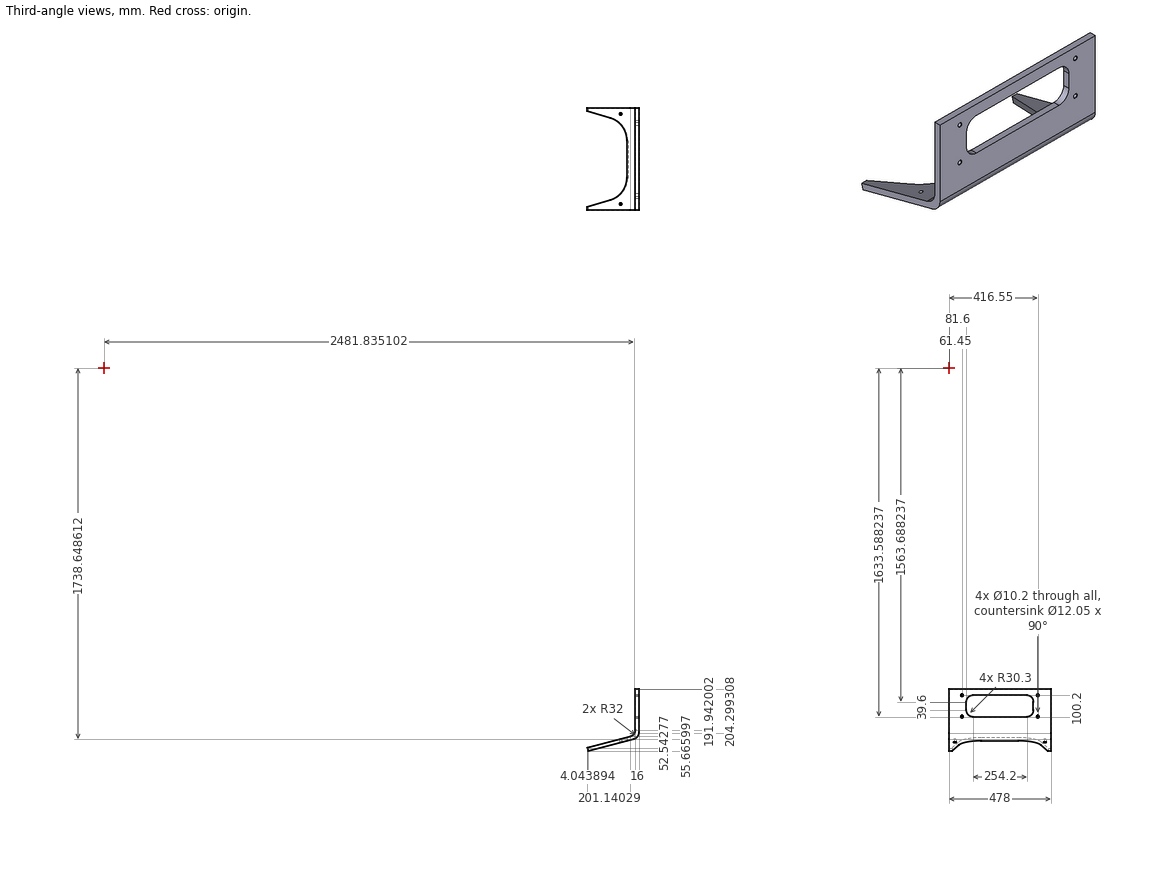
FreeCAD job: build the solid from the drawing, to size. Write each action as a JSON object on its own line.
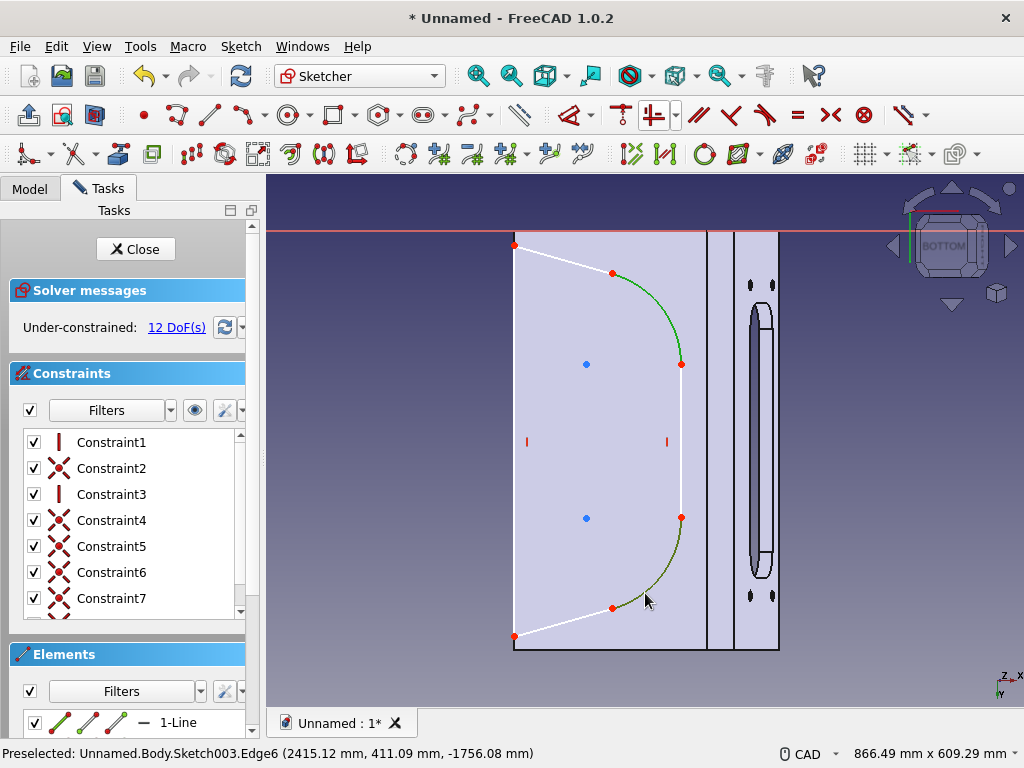
{"action": "left_click", "coordinate": [798, 116]}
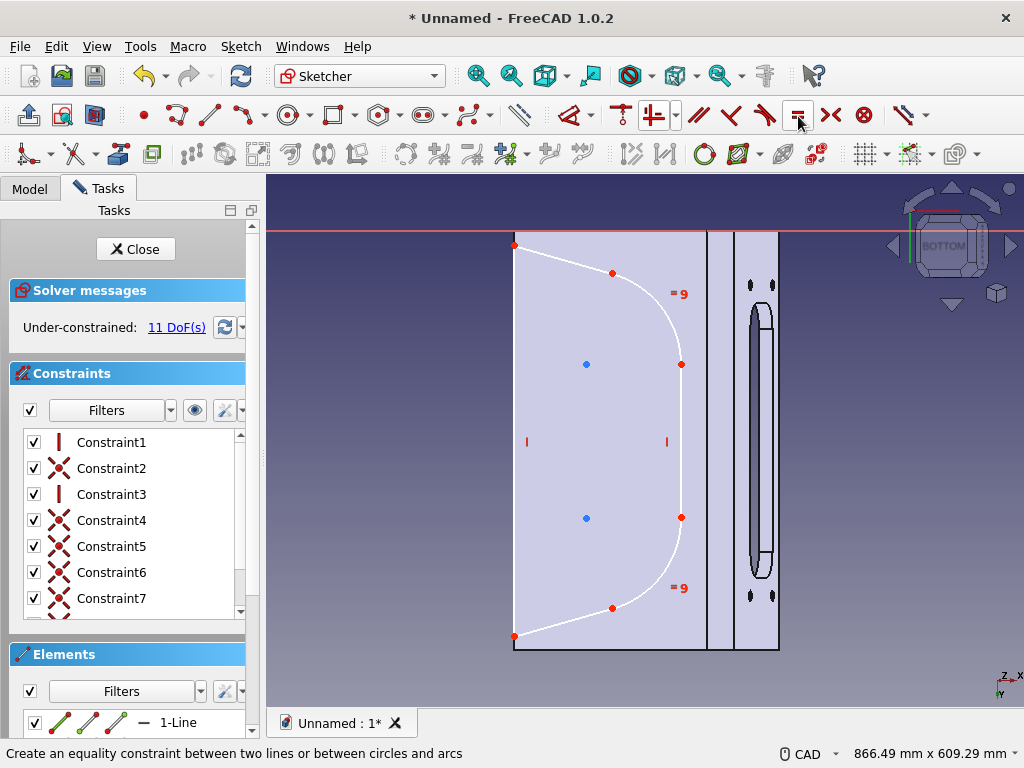
{"action": "left_click", "coordinate": [568, 116]}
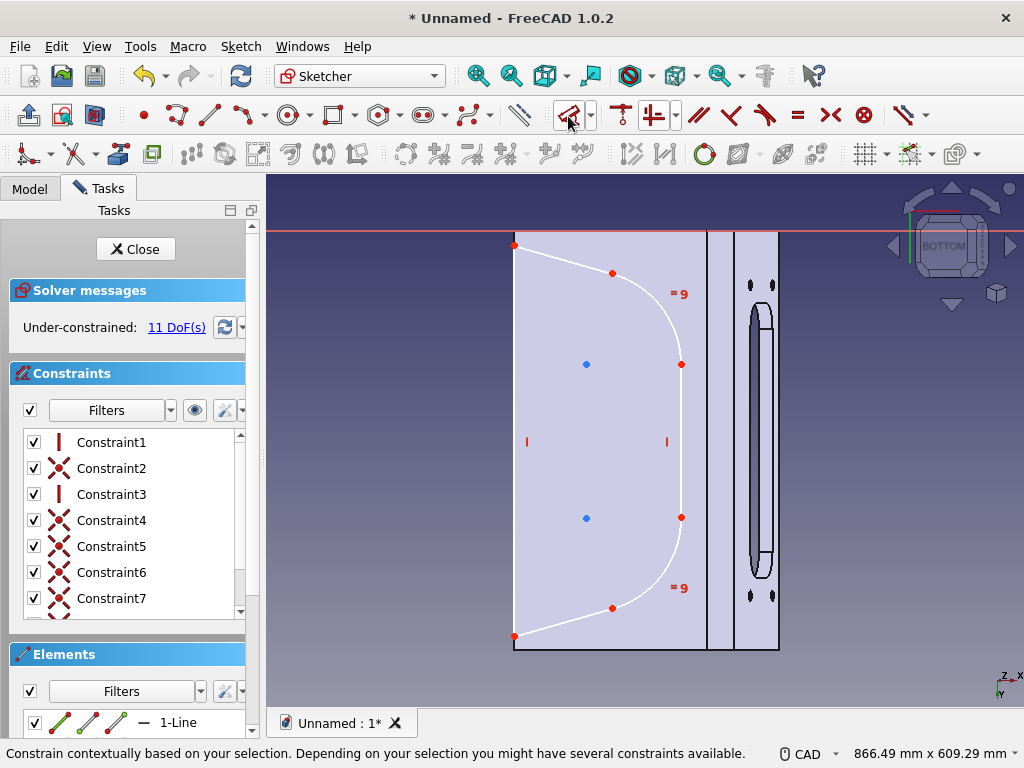
{"action": "left_click", "coordinate": [674, 329]}
{"action": "left_click", "coordinate": [704, 317]}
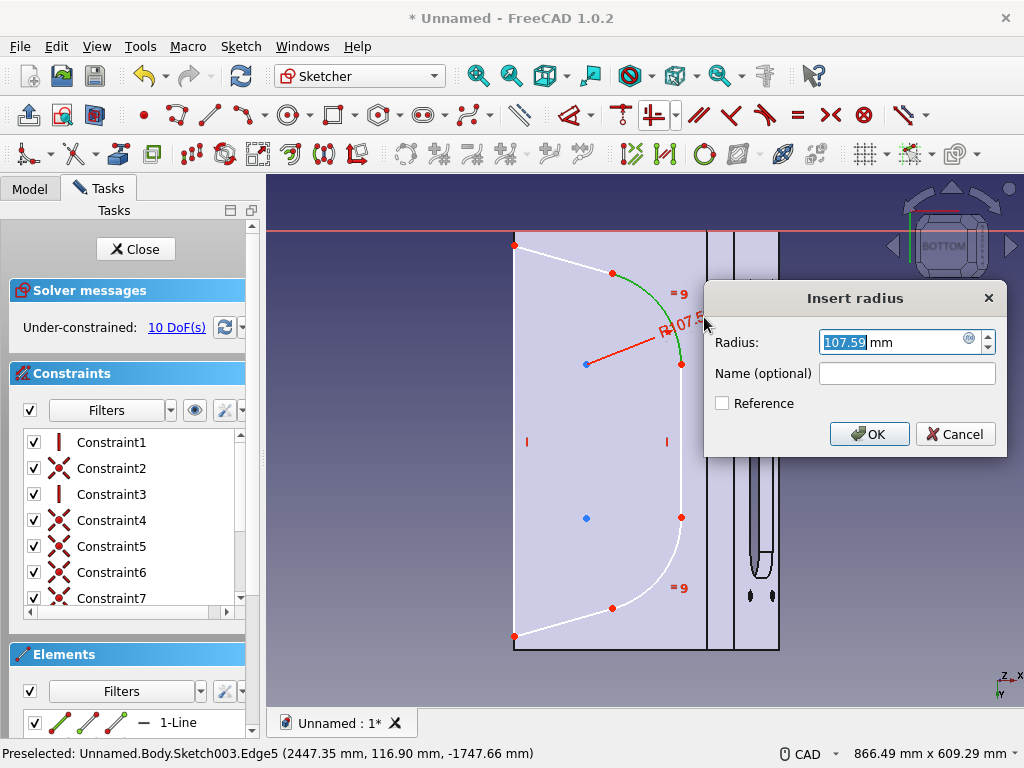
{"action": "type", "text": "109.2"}
{"action": "key", "text": "Return"}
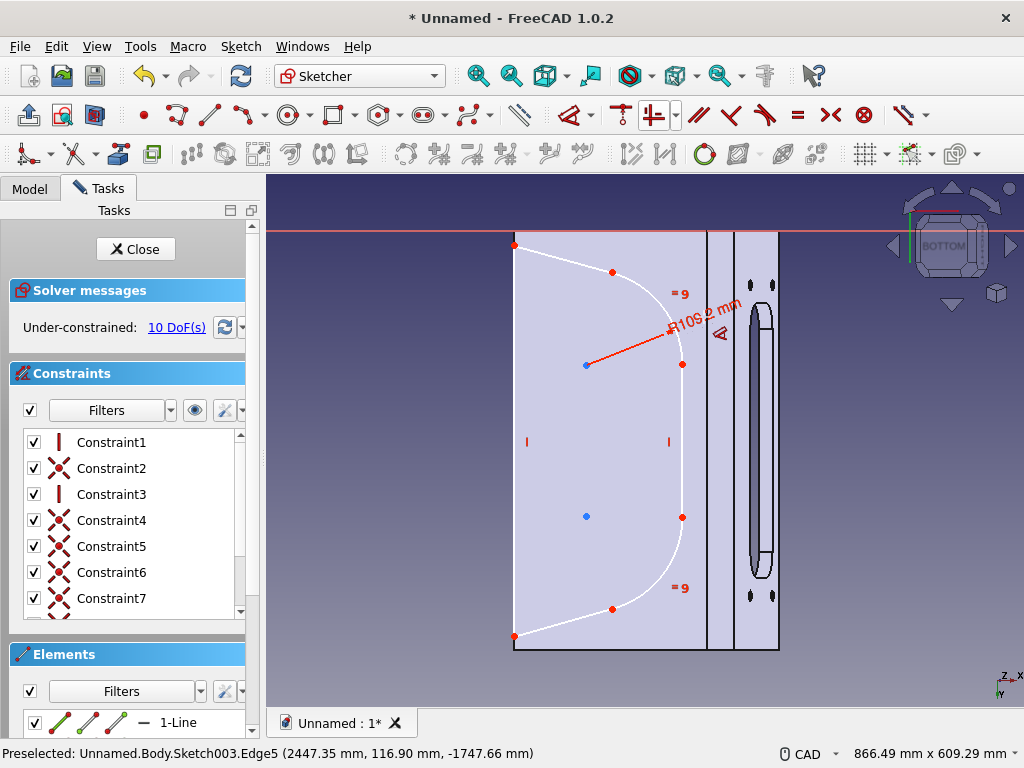
{"action": "left_click", "coordinate": [514, 363]}
{"action": "left_click", "coordinate": [480, 442]}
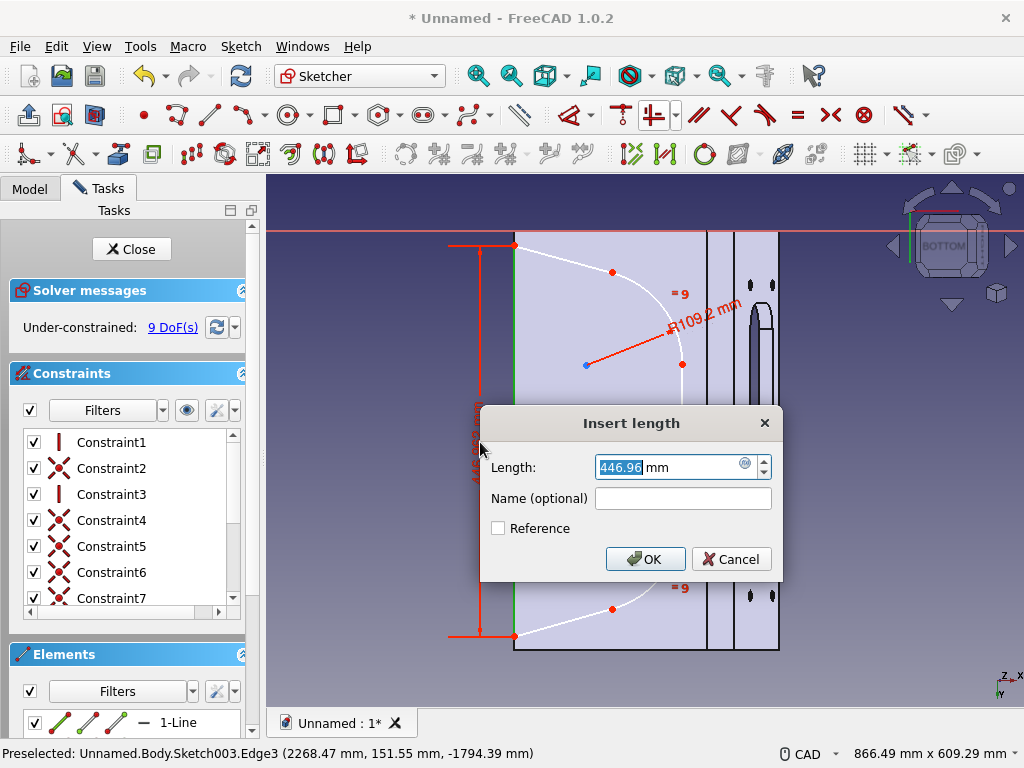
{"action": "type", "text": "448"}
{"action": "key", "text": "Return"}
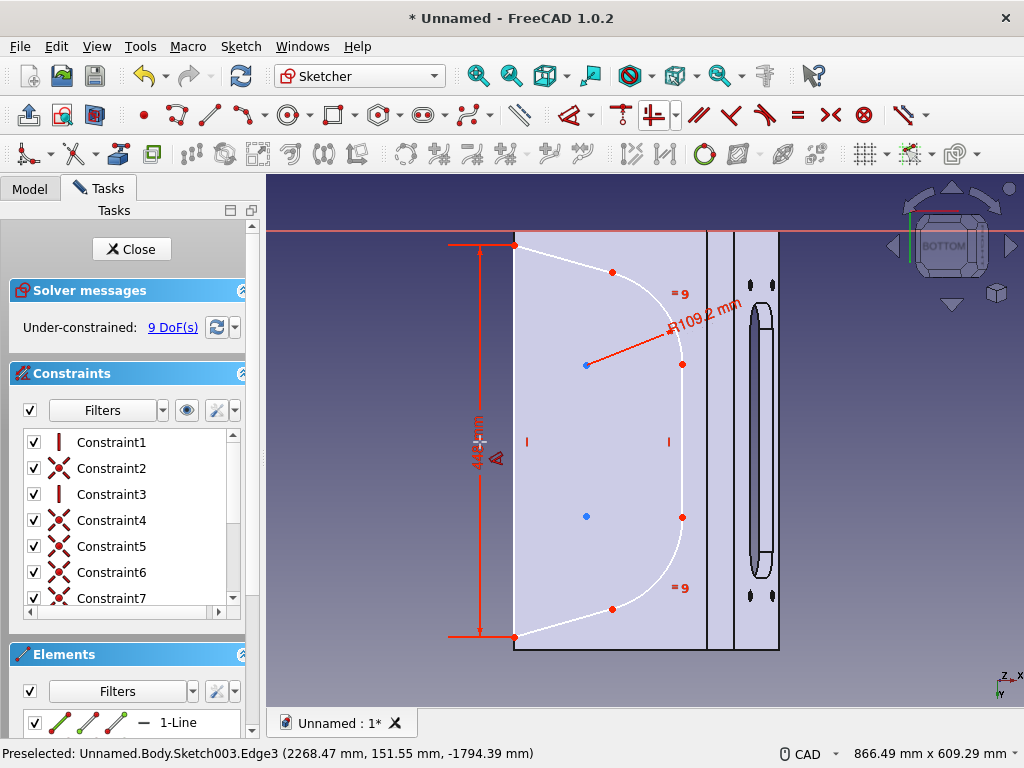
{"action": "scroll", "coordinate": [514, 245], "scroll_direction": "up", "scroll_amount": 6}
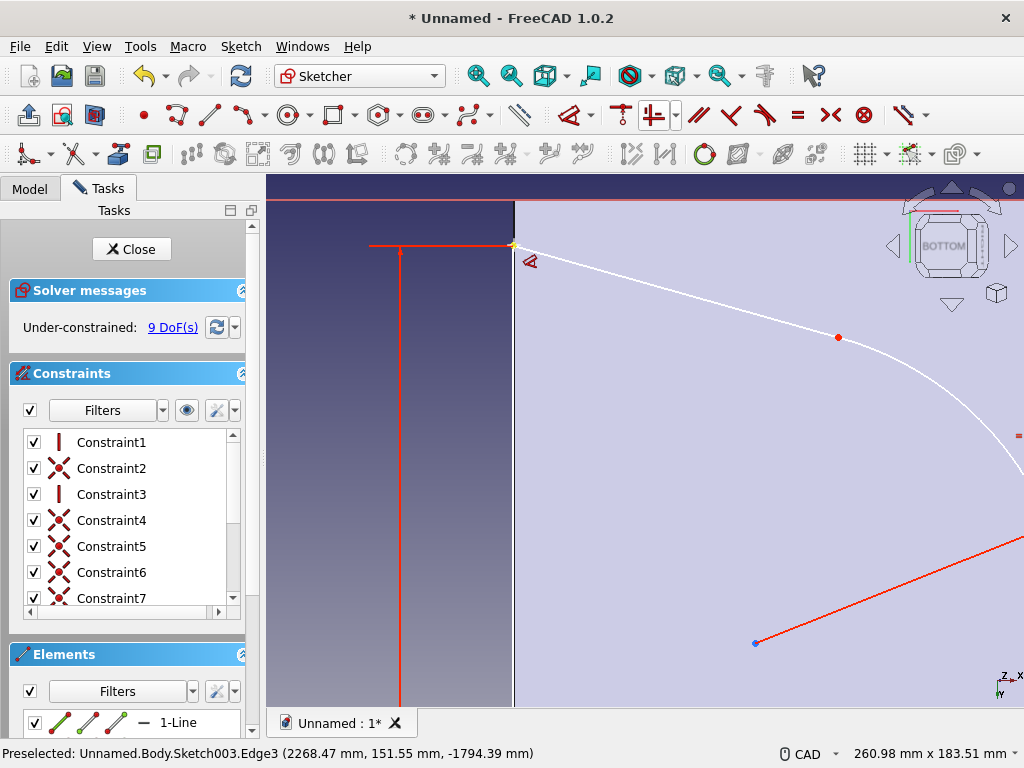
{"action": "left_click", "coordinate": [513, 246]}
{"action": "left_click", "coordinate": [547, 224]}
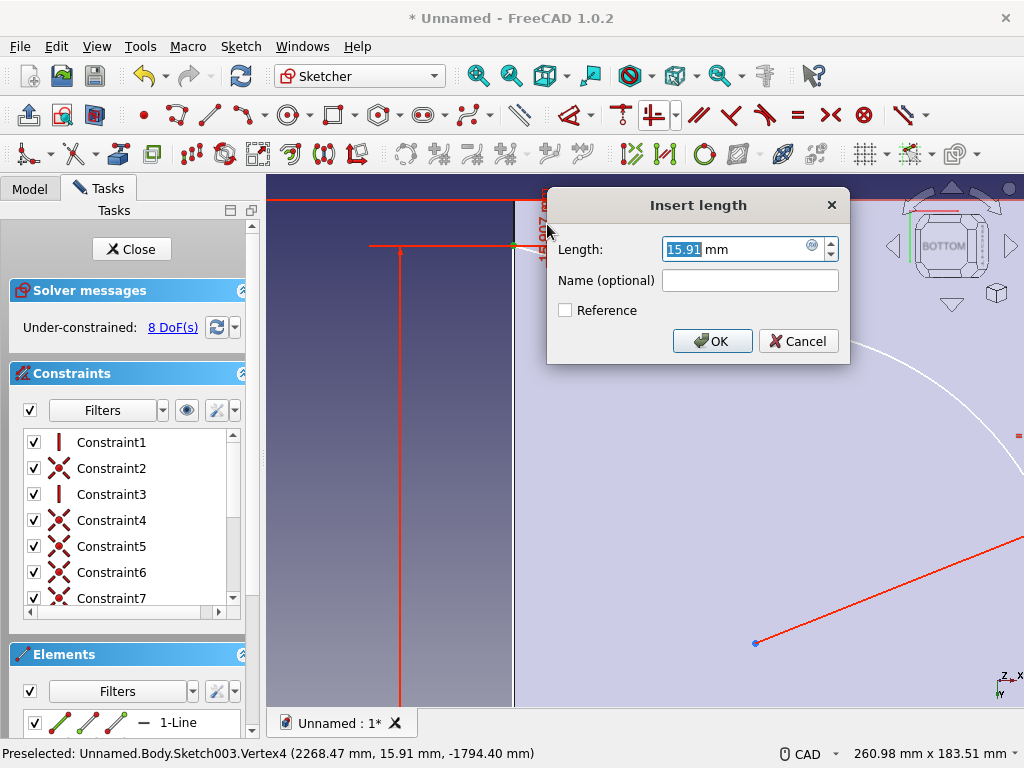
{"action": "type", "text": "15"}
{"action": "key", "text": "Return"}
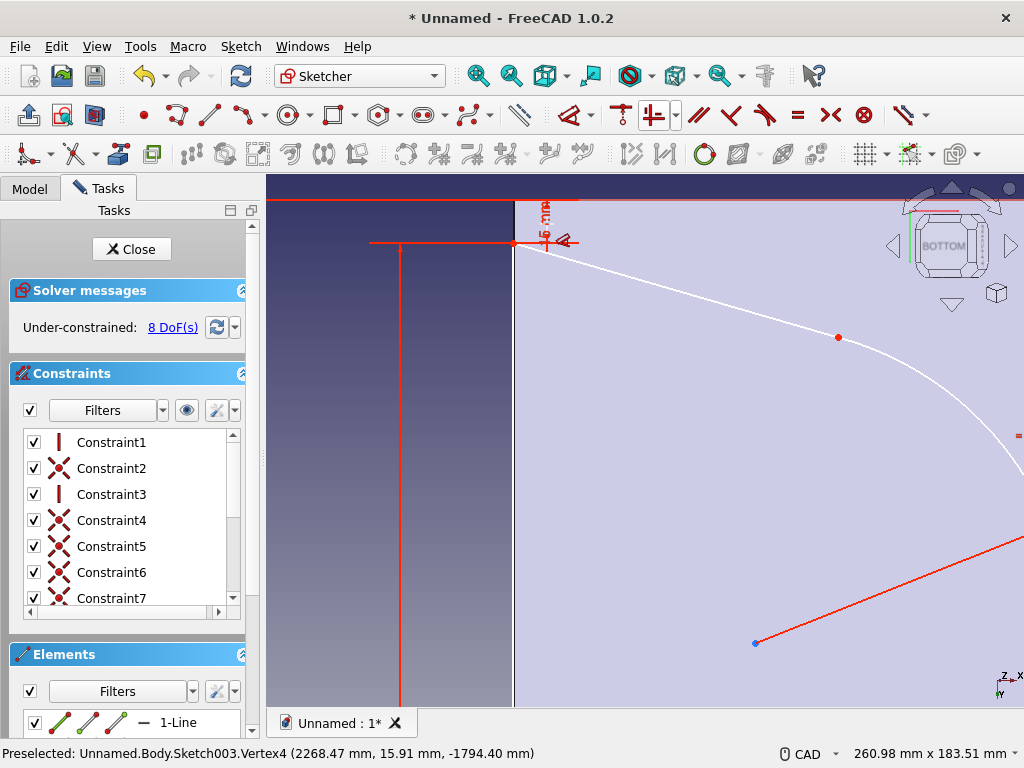
{"action": "scroll", "coordinate": [506, 292], "scroll_direction": "down", "scroll_amount": 7}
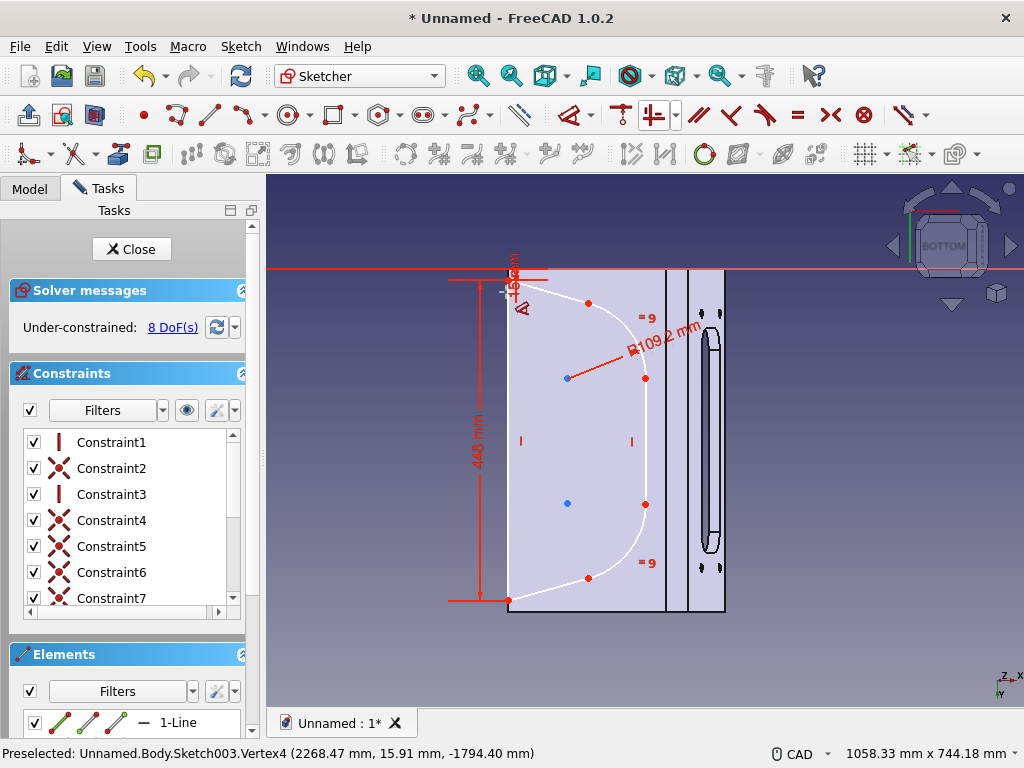
{"action": "left_click", "coordinate": [646, 466]}
{"action": "left_click", "coordinate": [680, 441]}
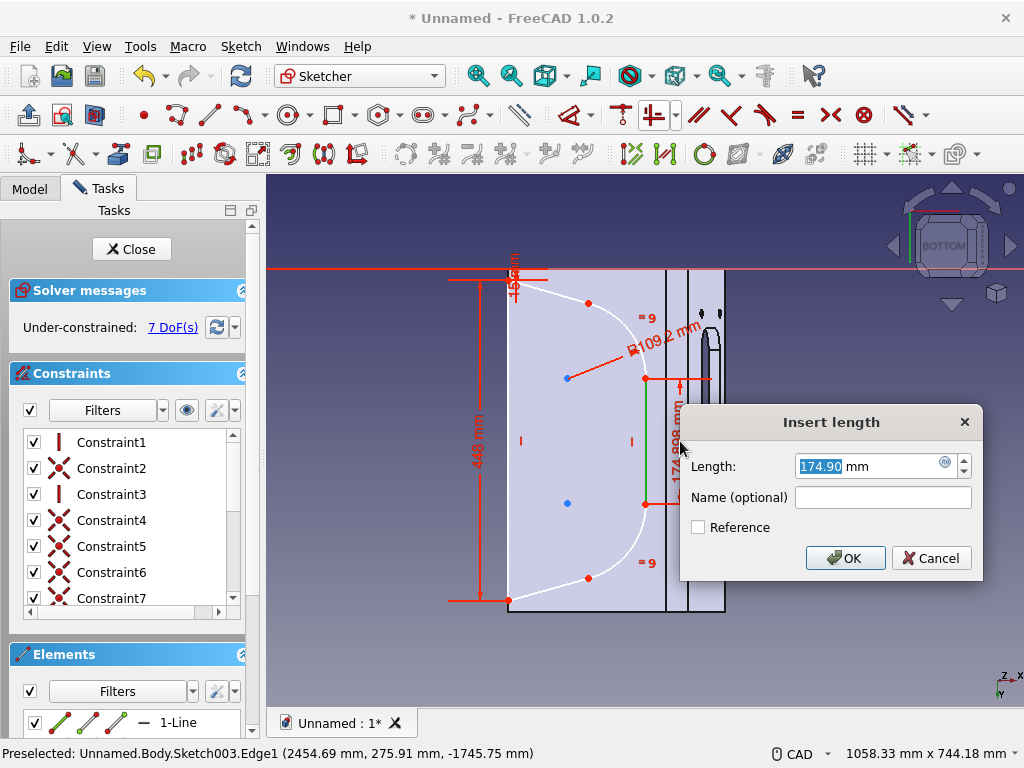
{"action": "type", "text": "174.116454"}
{"action": "key", "text": "Return"}